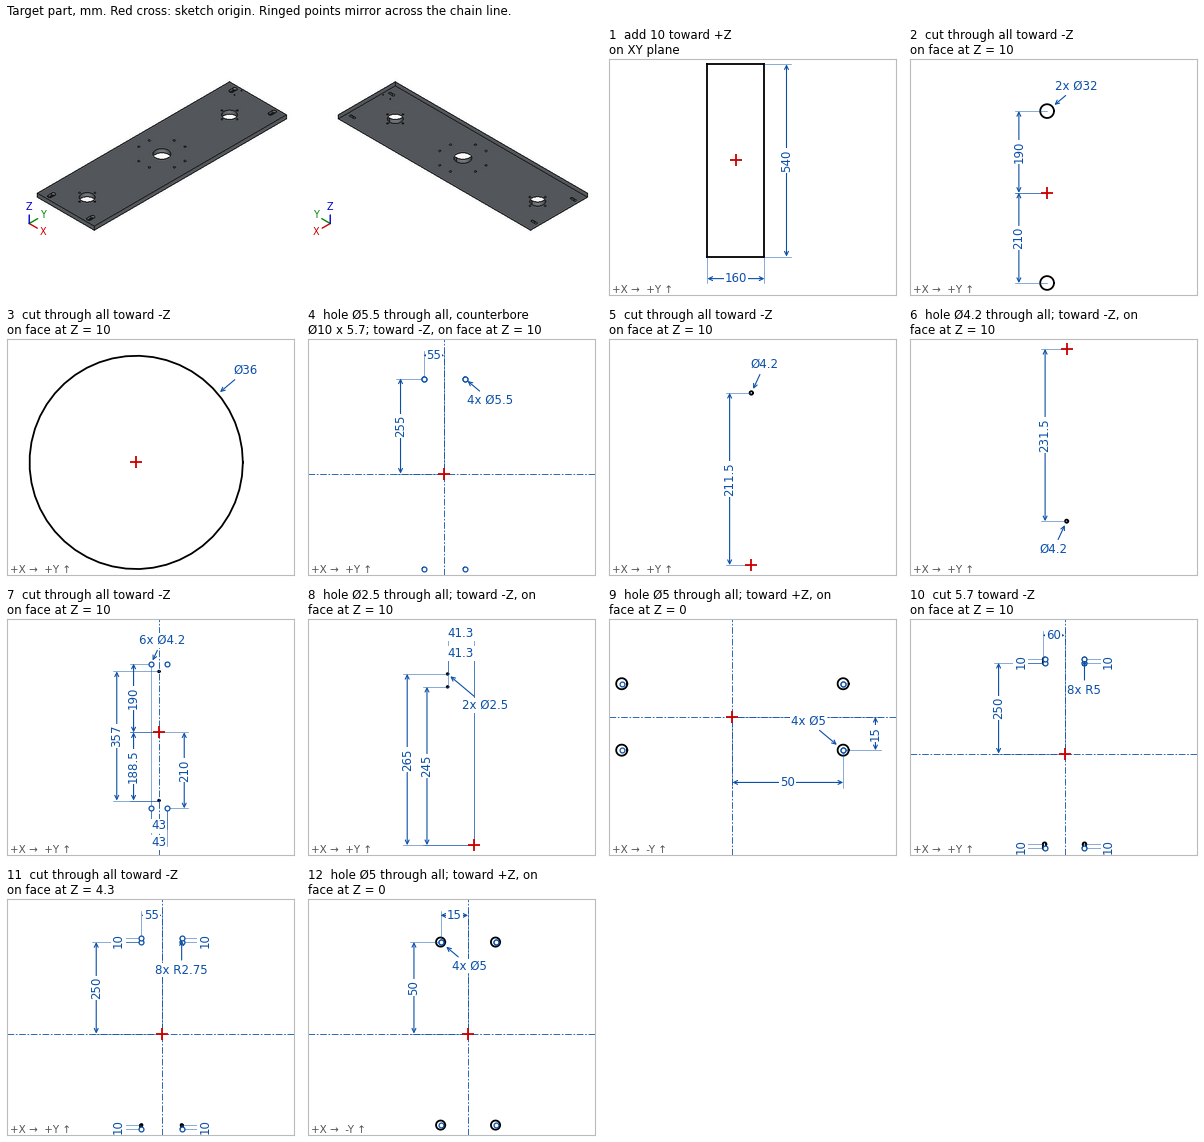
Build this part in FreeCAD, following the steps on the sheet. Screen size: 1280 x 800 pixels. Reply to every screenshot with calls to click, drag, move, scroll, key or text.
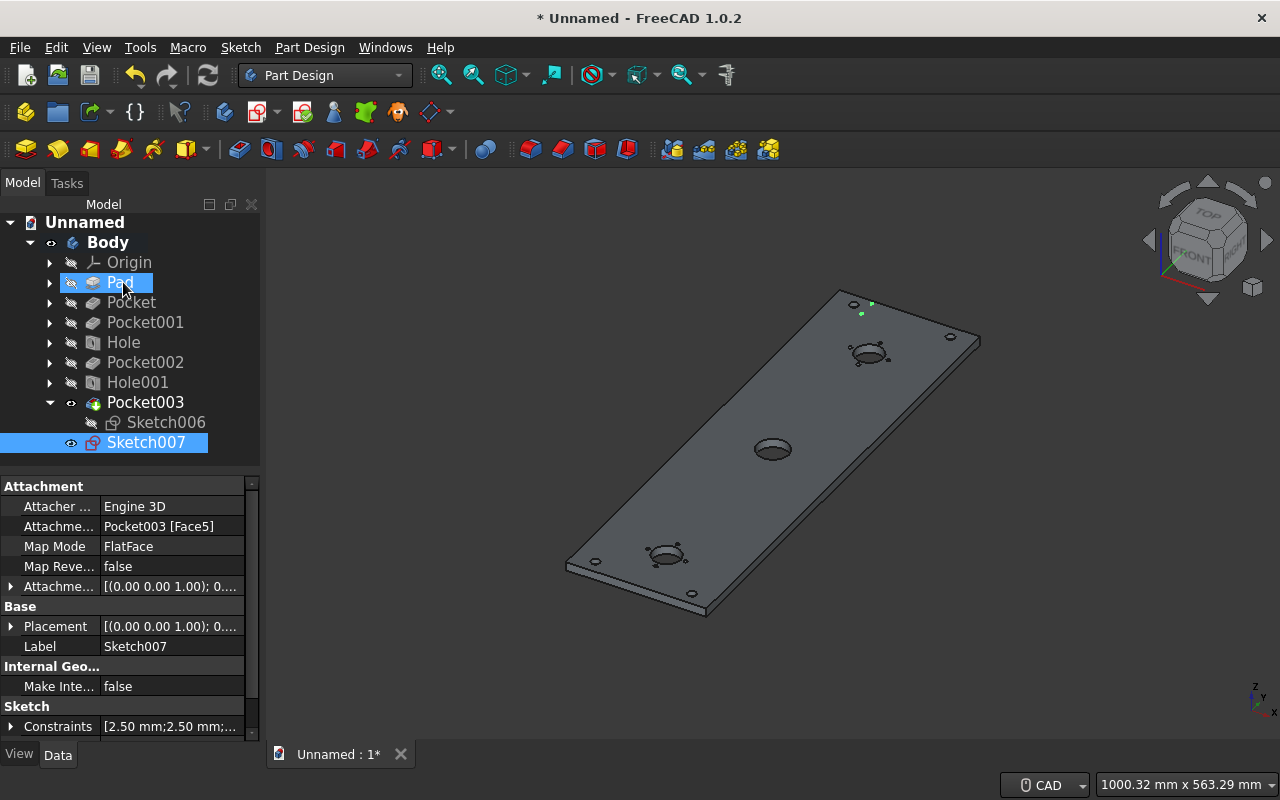
click(272, 150)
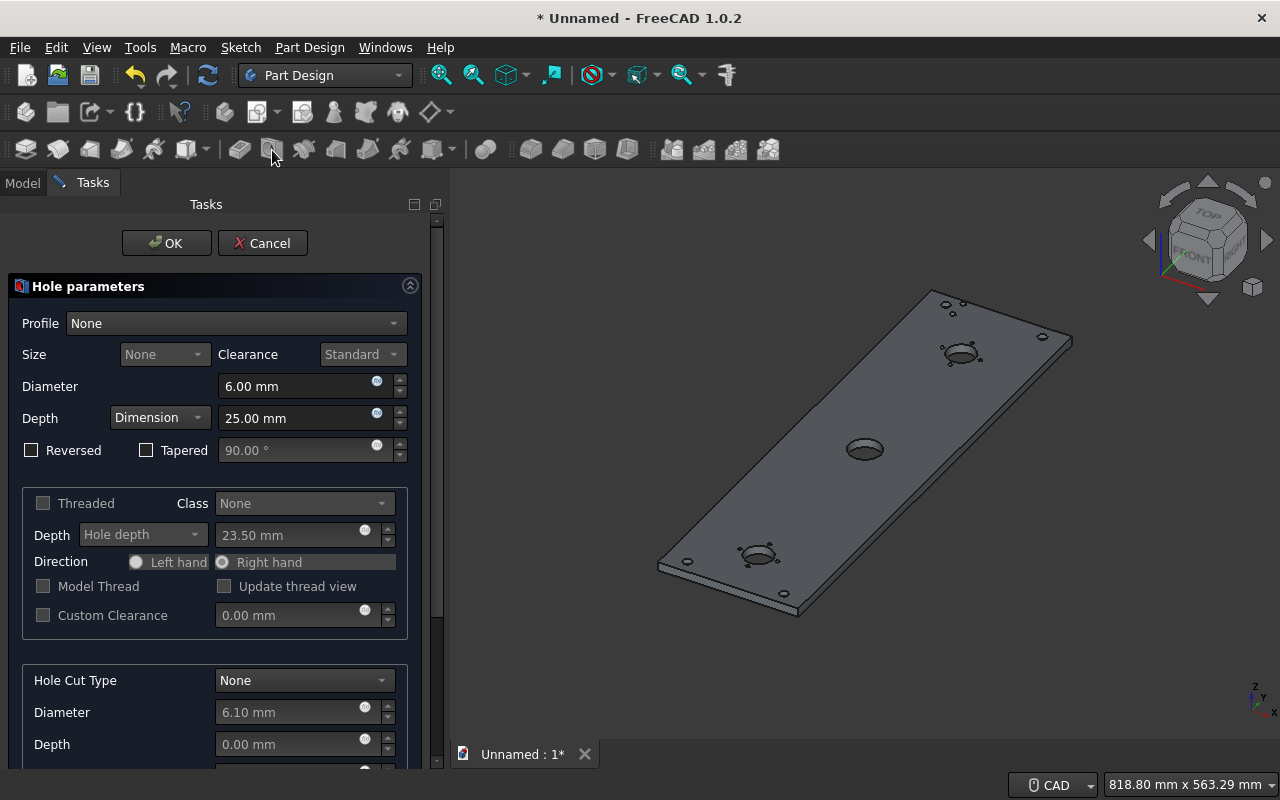
triple_click(305, 386)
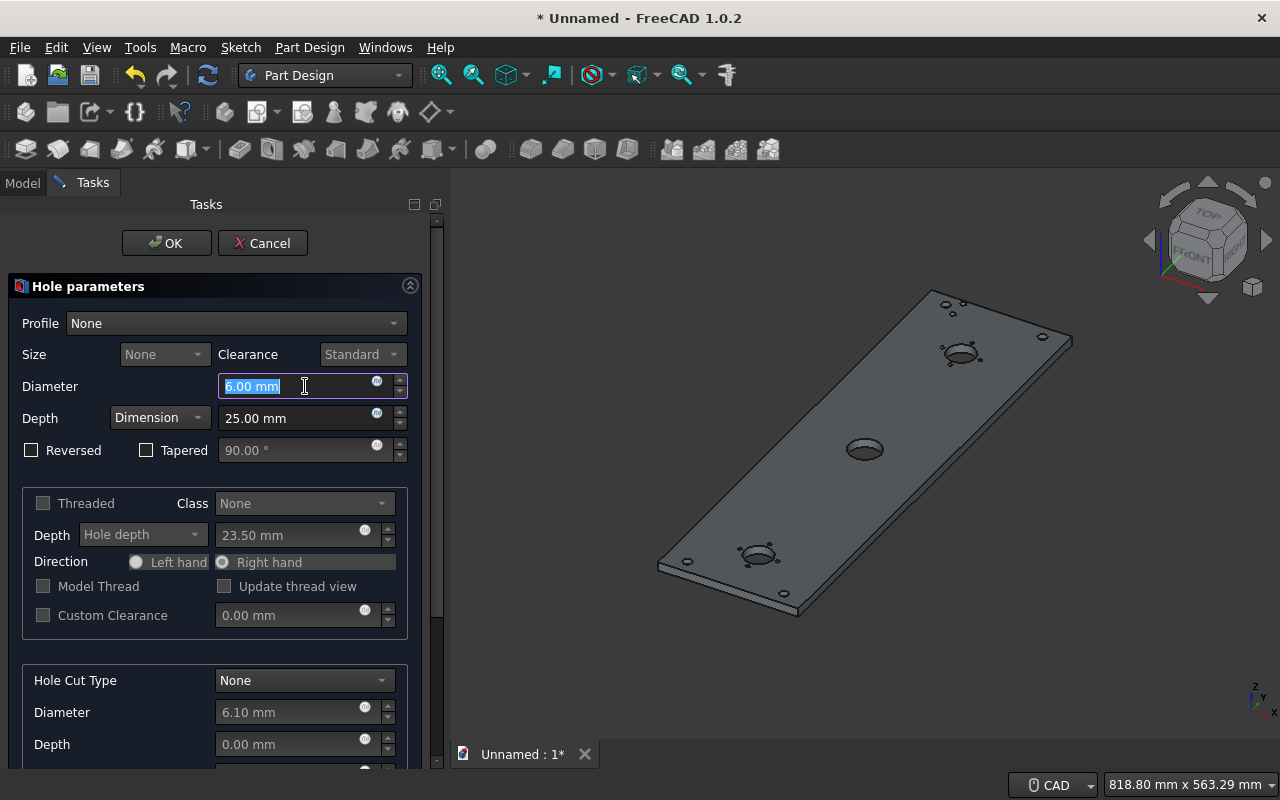
text(2.5)
key(Tab)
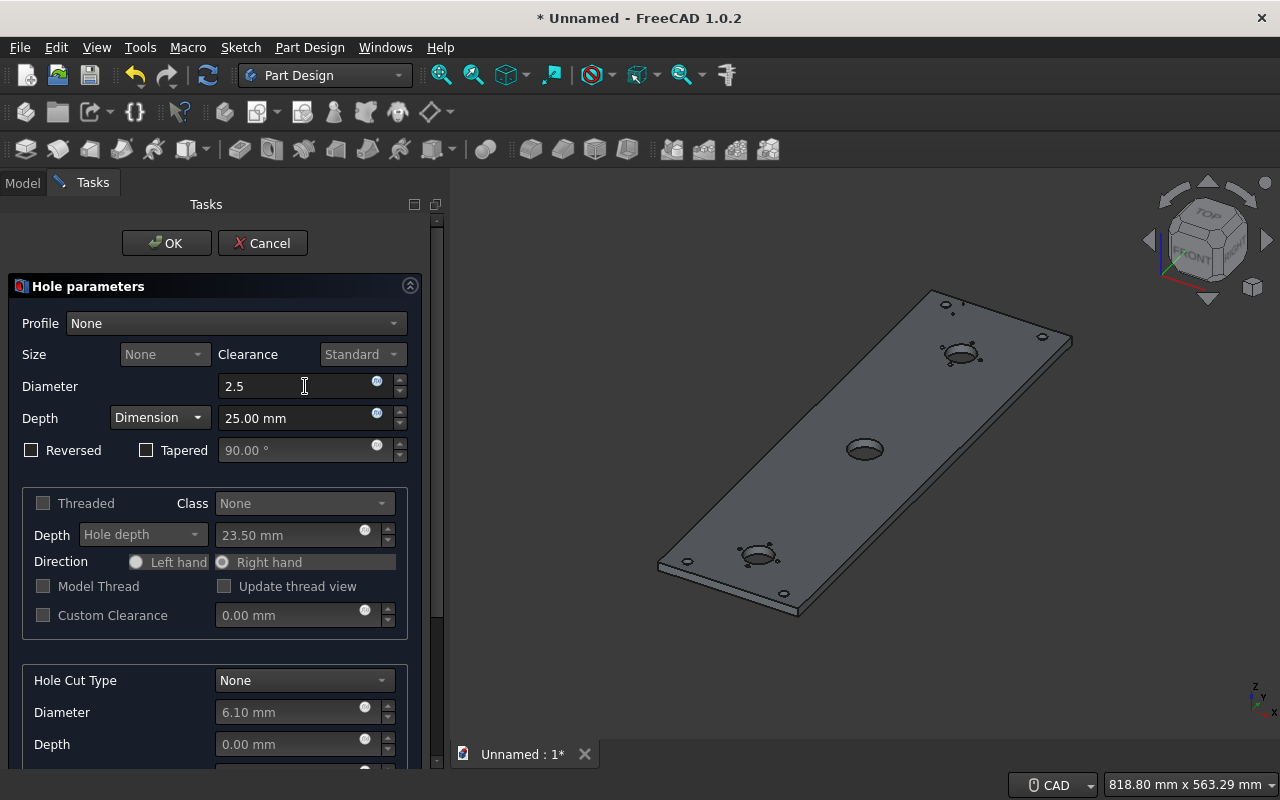
click(161, 418)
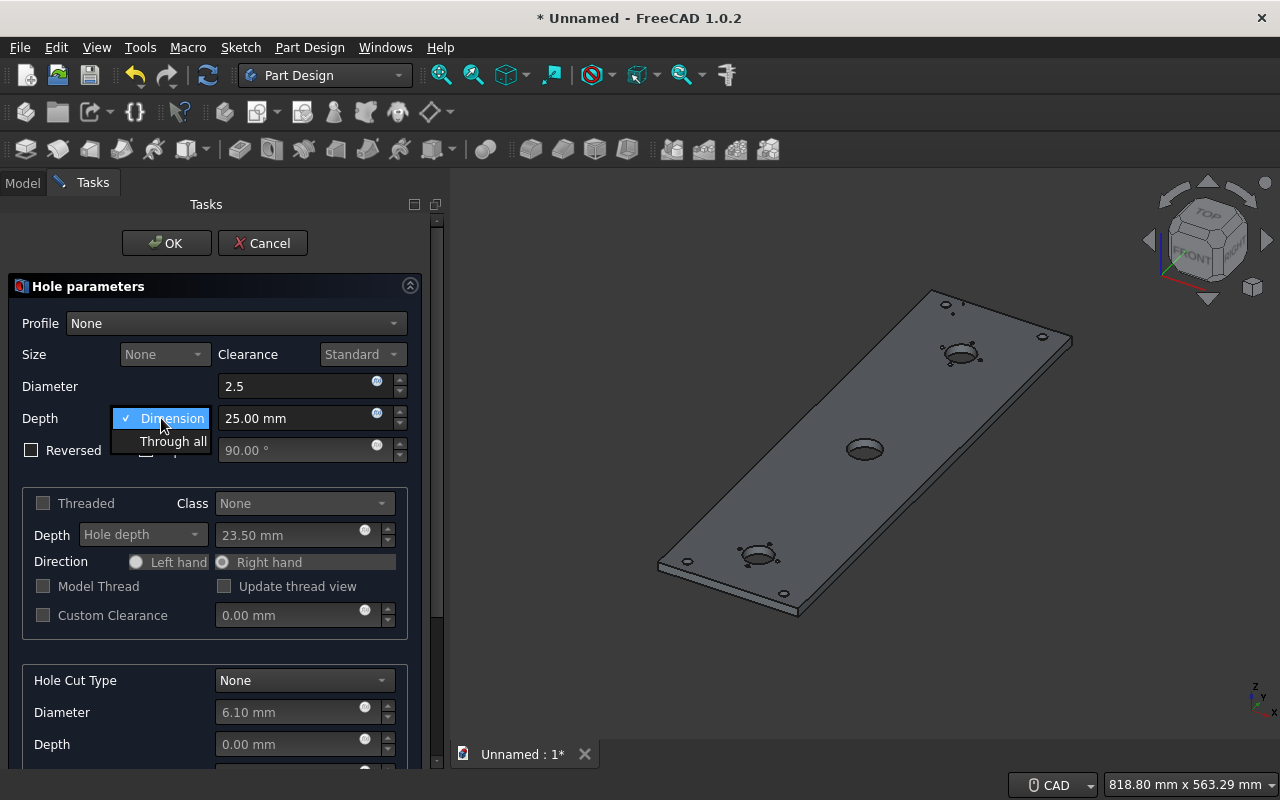
click(160, 442)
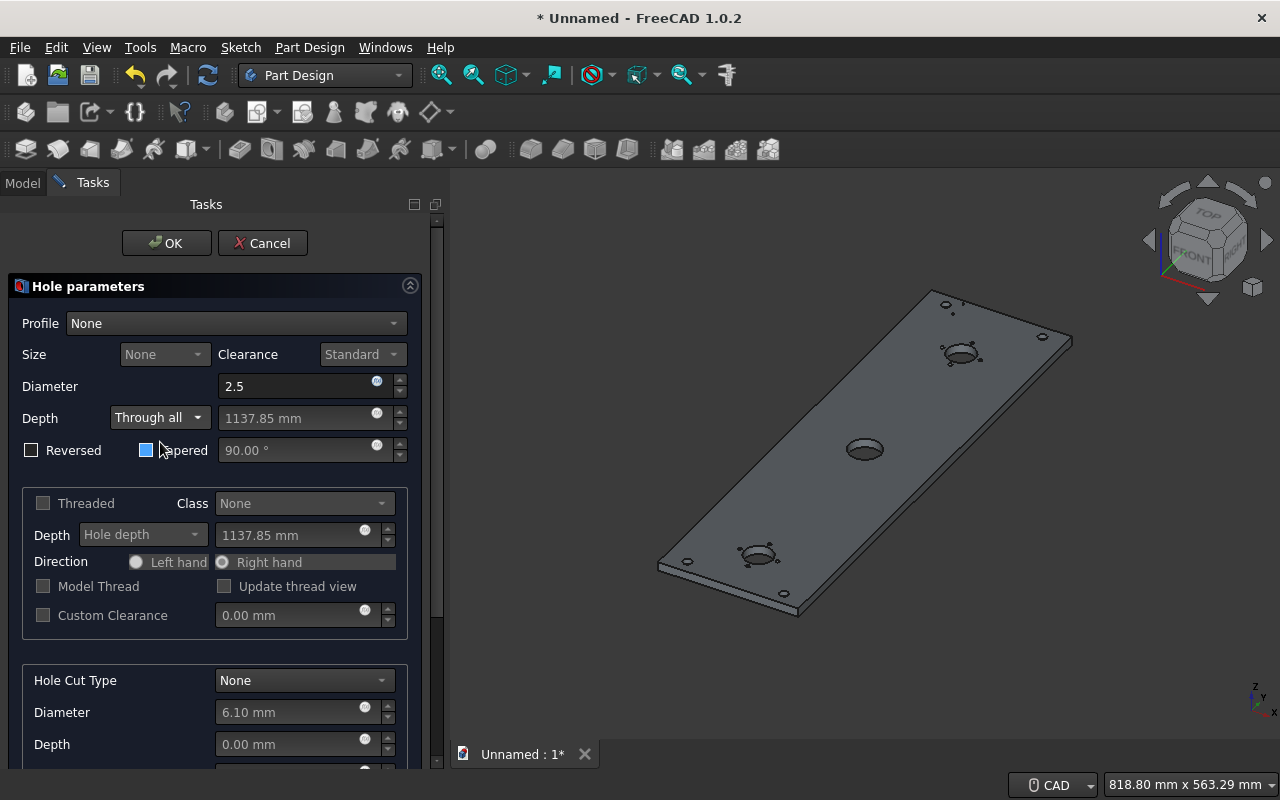
click(167, 243)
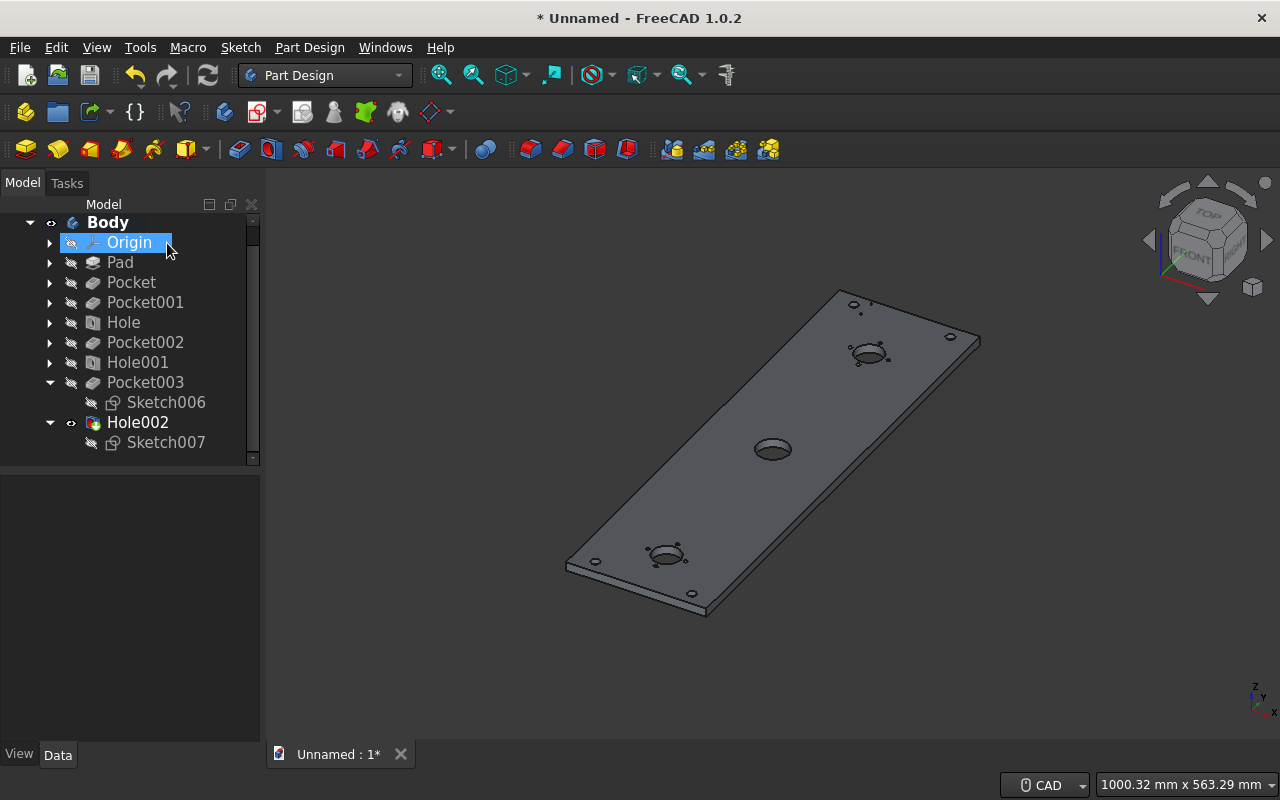
key(5)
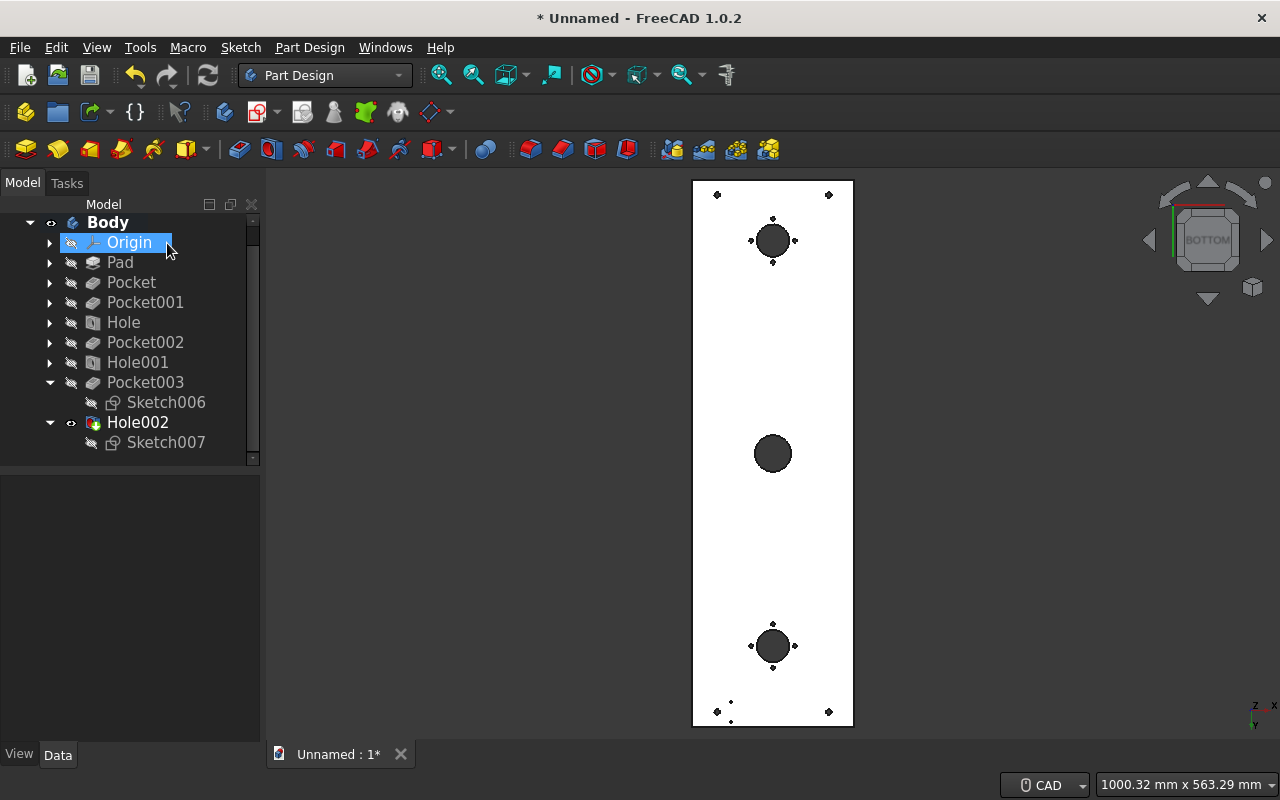
click(773, 531)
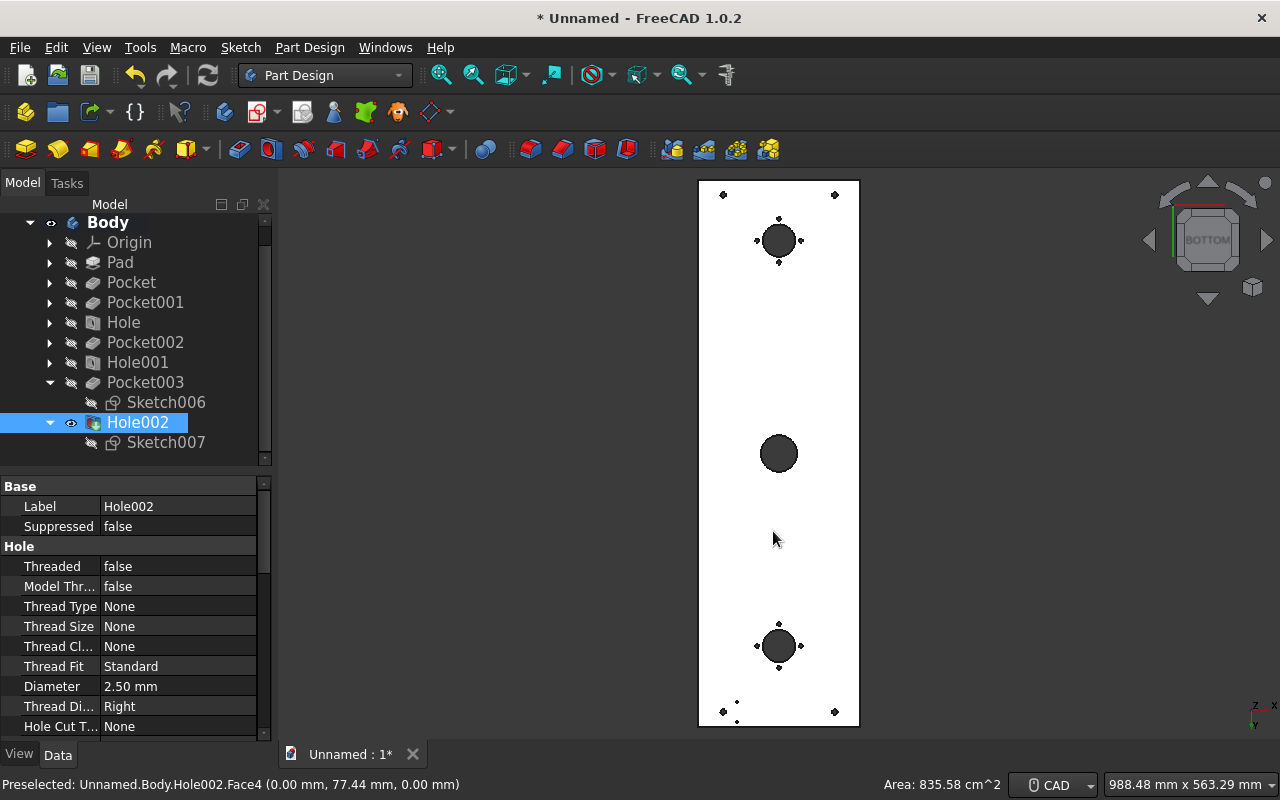
click(258, 112)